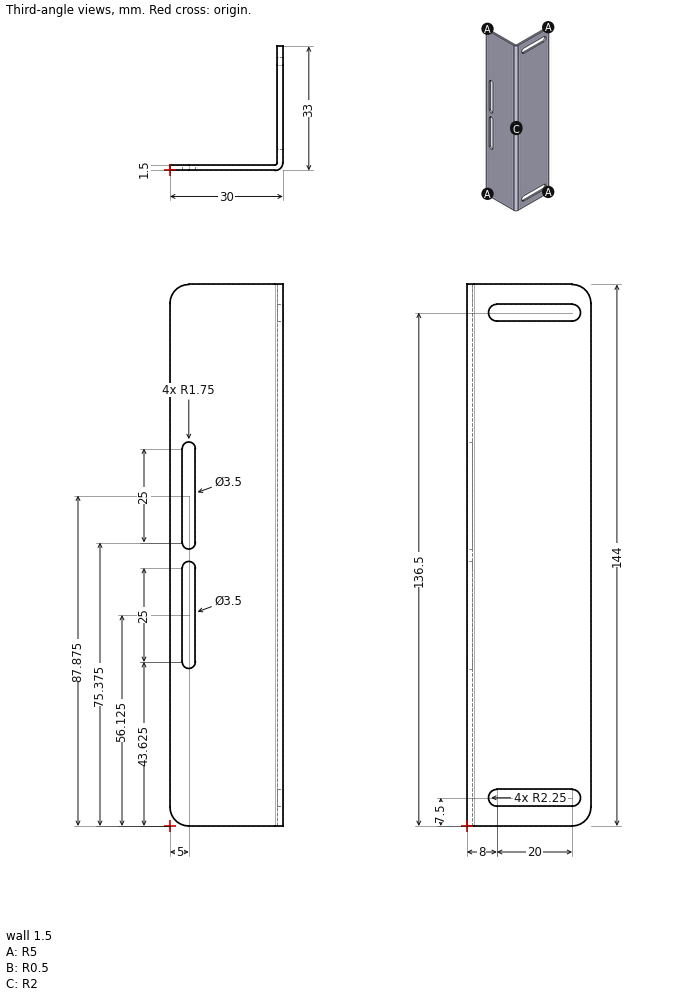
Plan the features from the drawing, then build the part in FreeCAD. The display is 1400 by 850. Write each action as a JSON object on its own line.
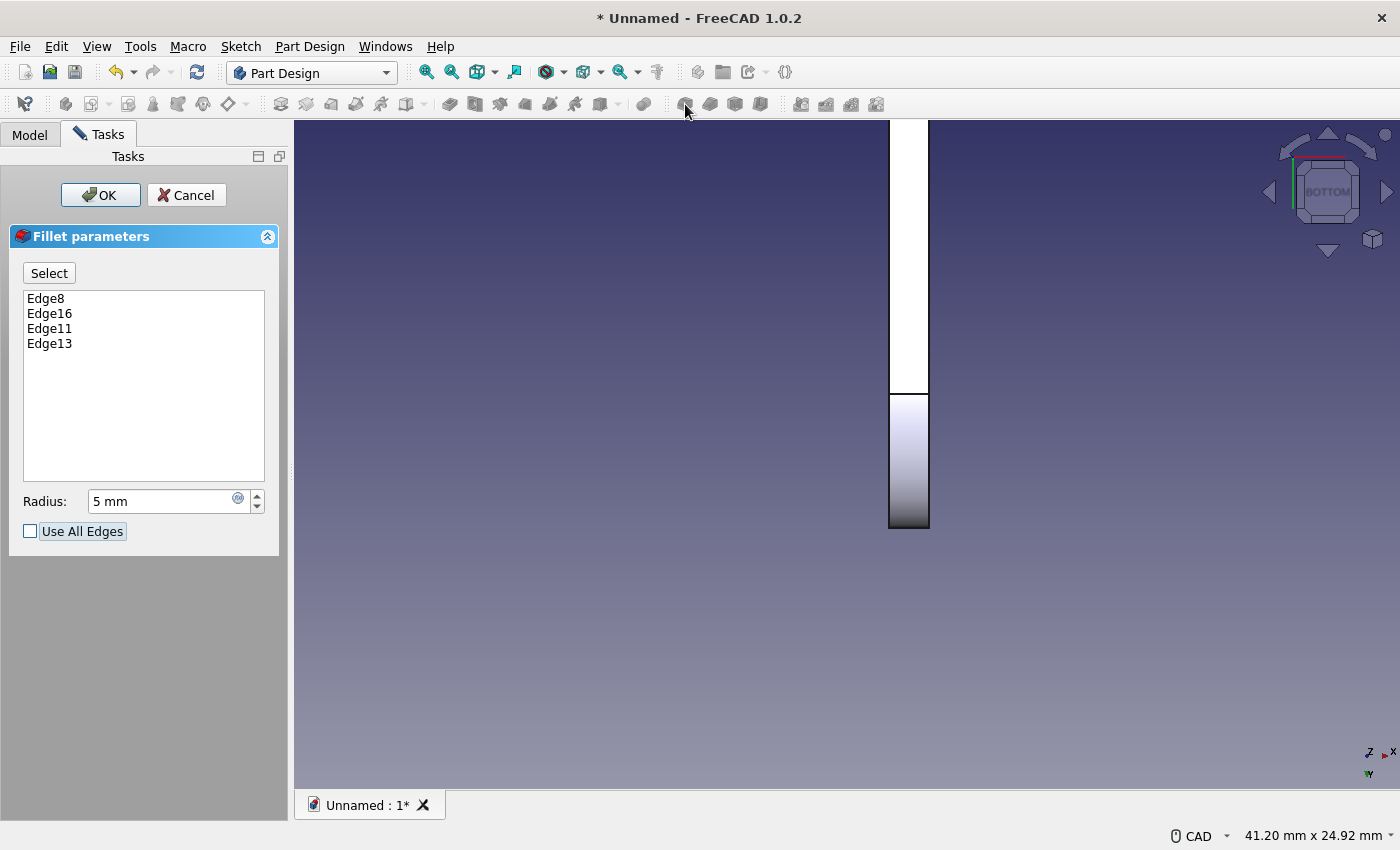
{"action": "left_click", "coordinate": [101, 195]}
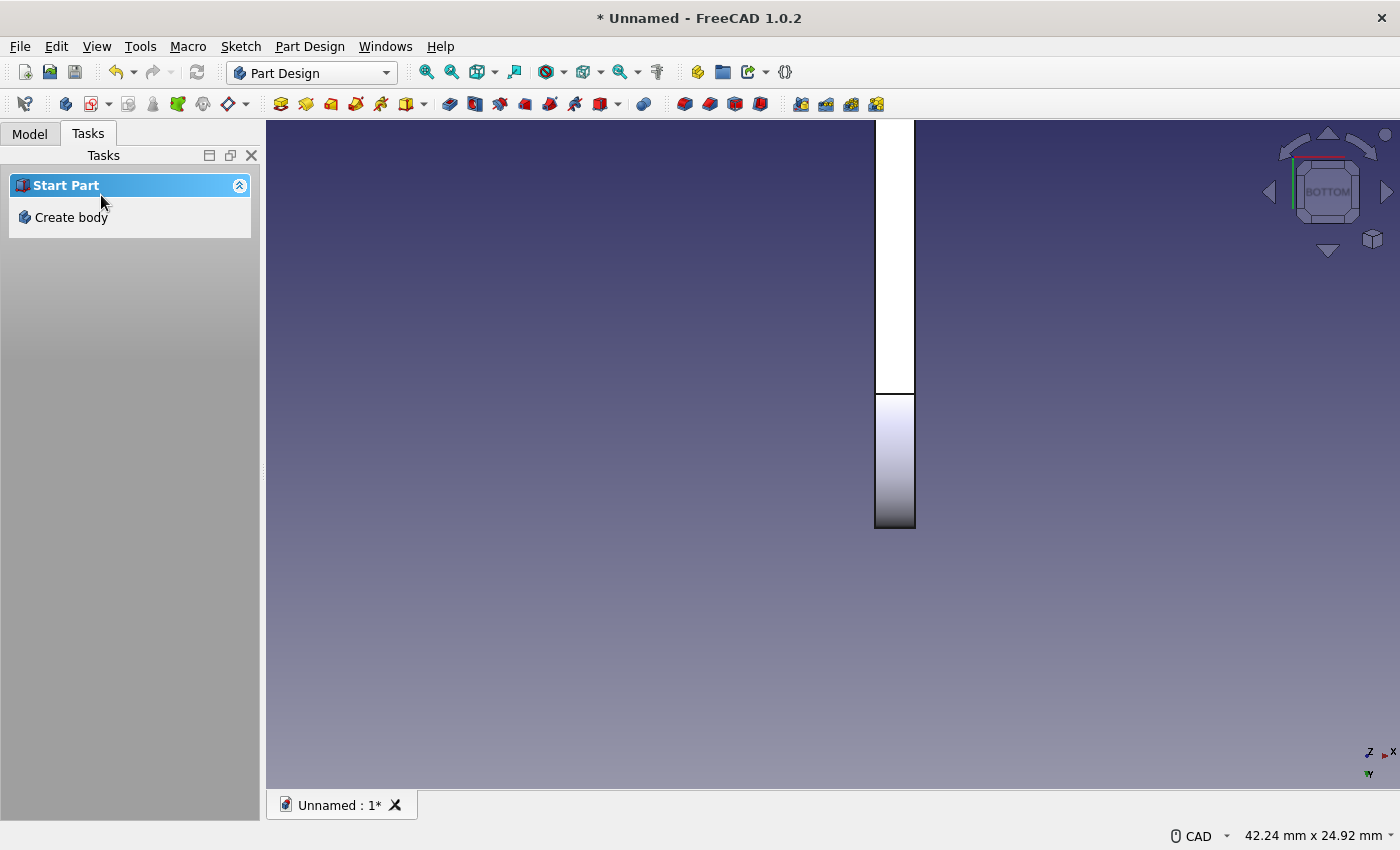
{"action": "left_click", "coordinate": [427, 72]}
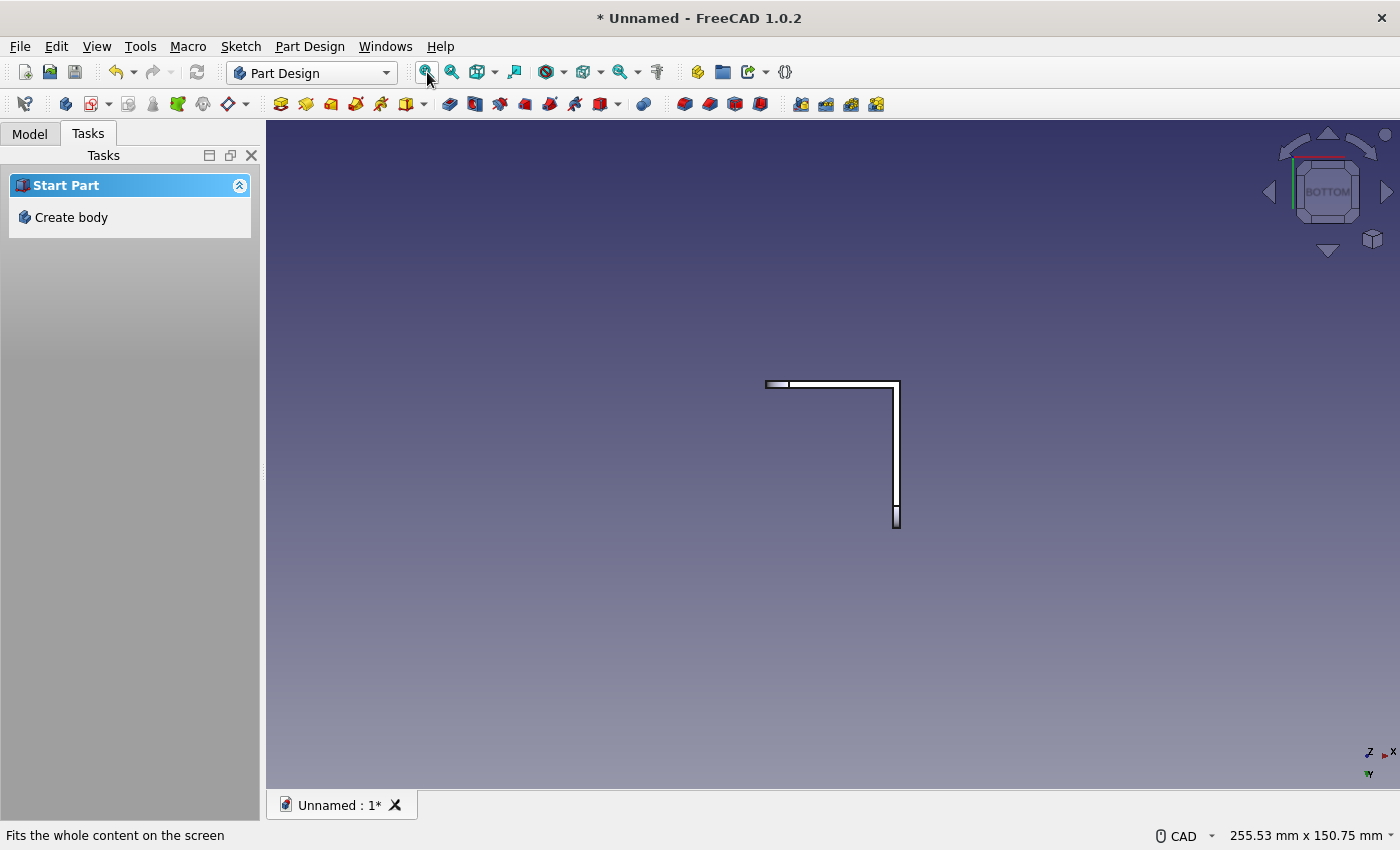
{"action": "key", "text": "0"}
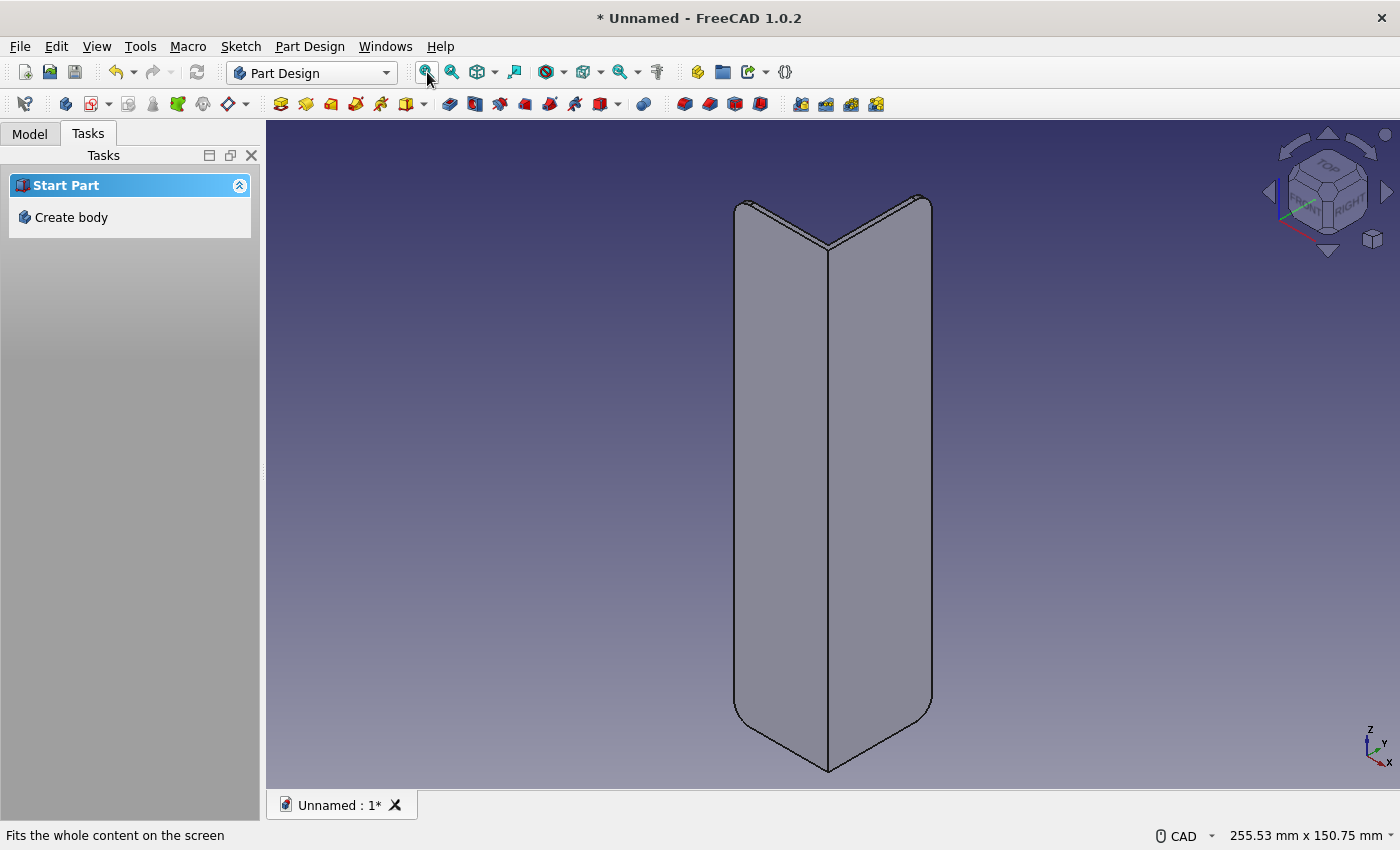
{"action": "key", "text": "2"}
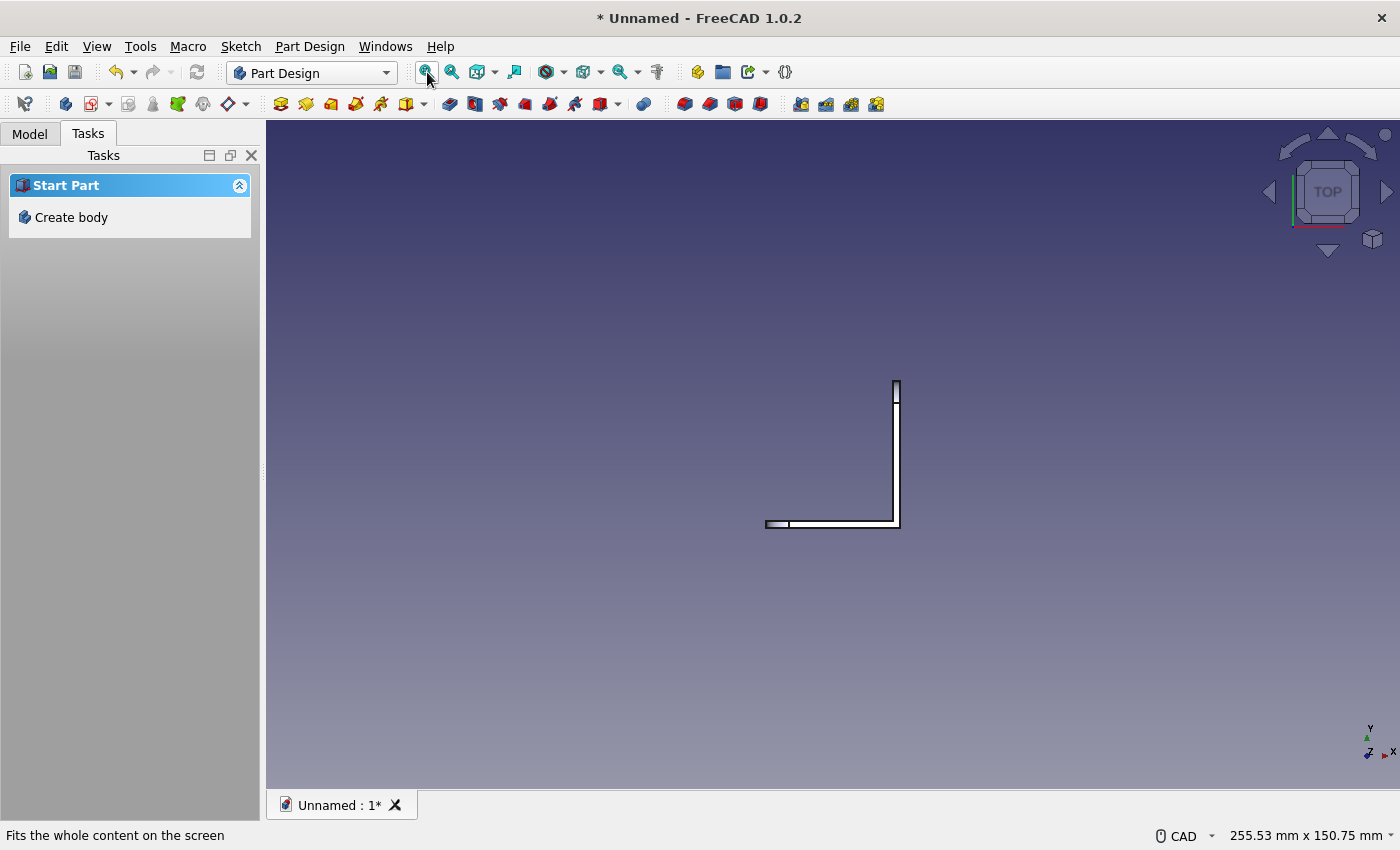
{"action": "left_click", "coordinate": [427, 72]}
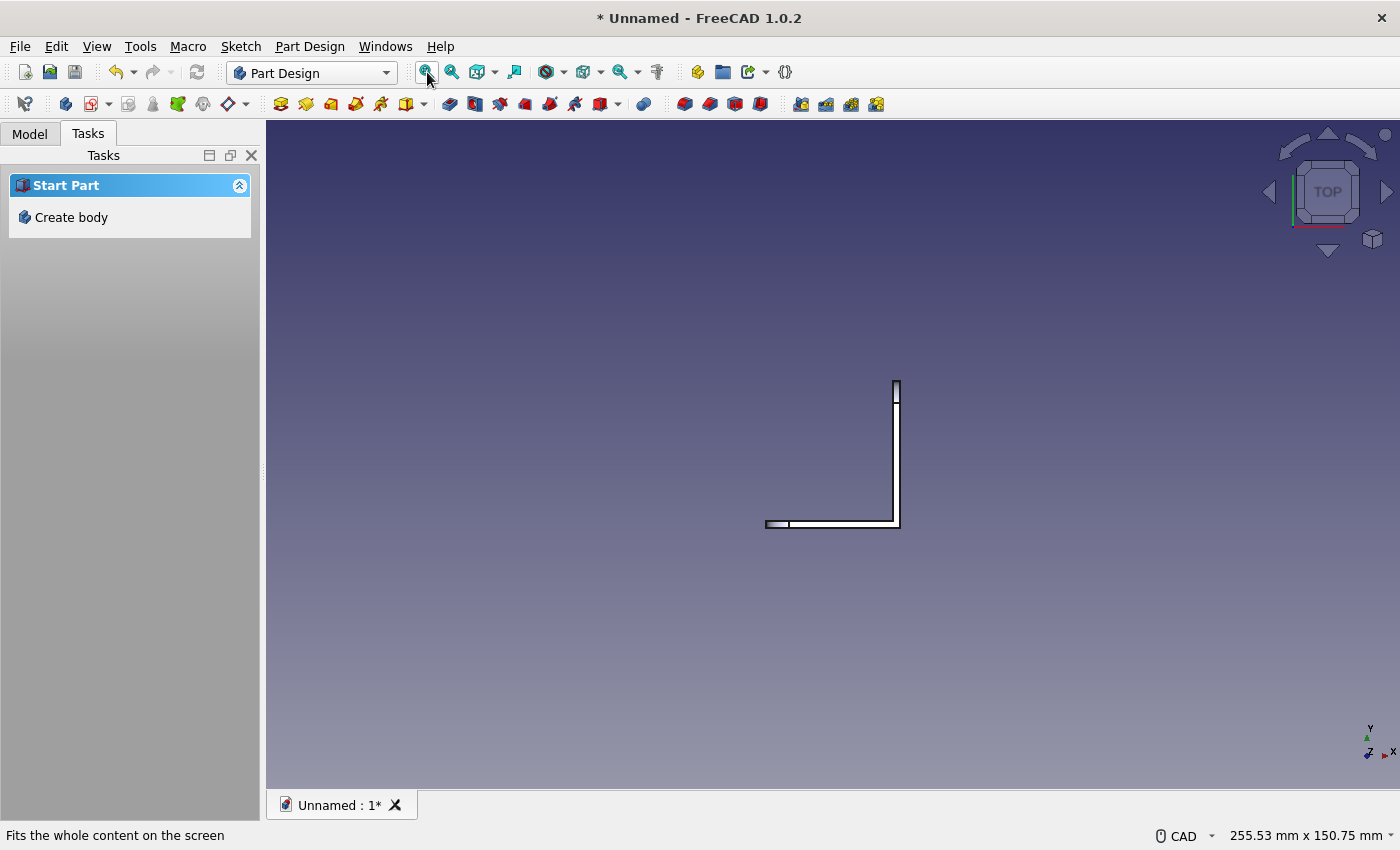
{"action": "key", "text": "1"}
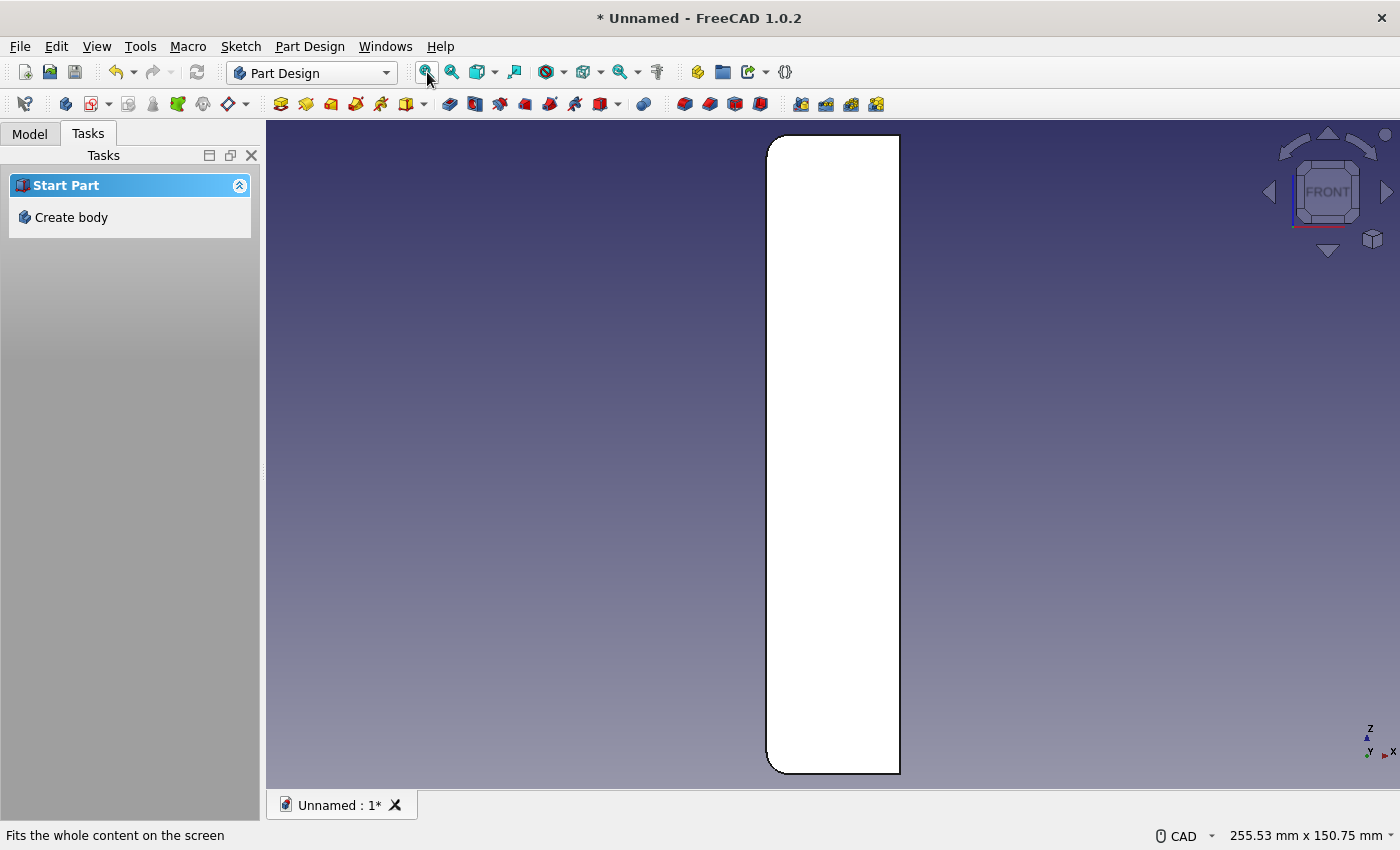
{"action": "key", "text": "3"}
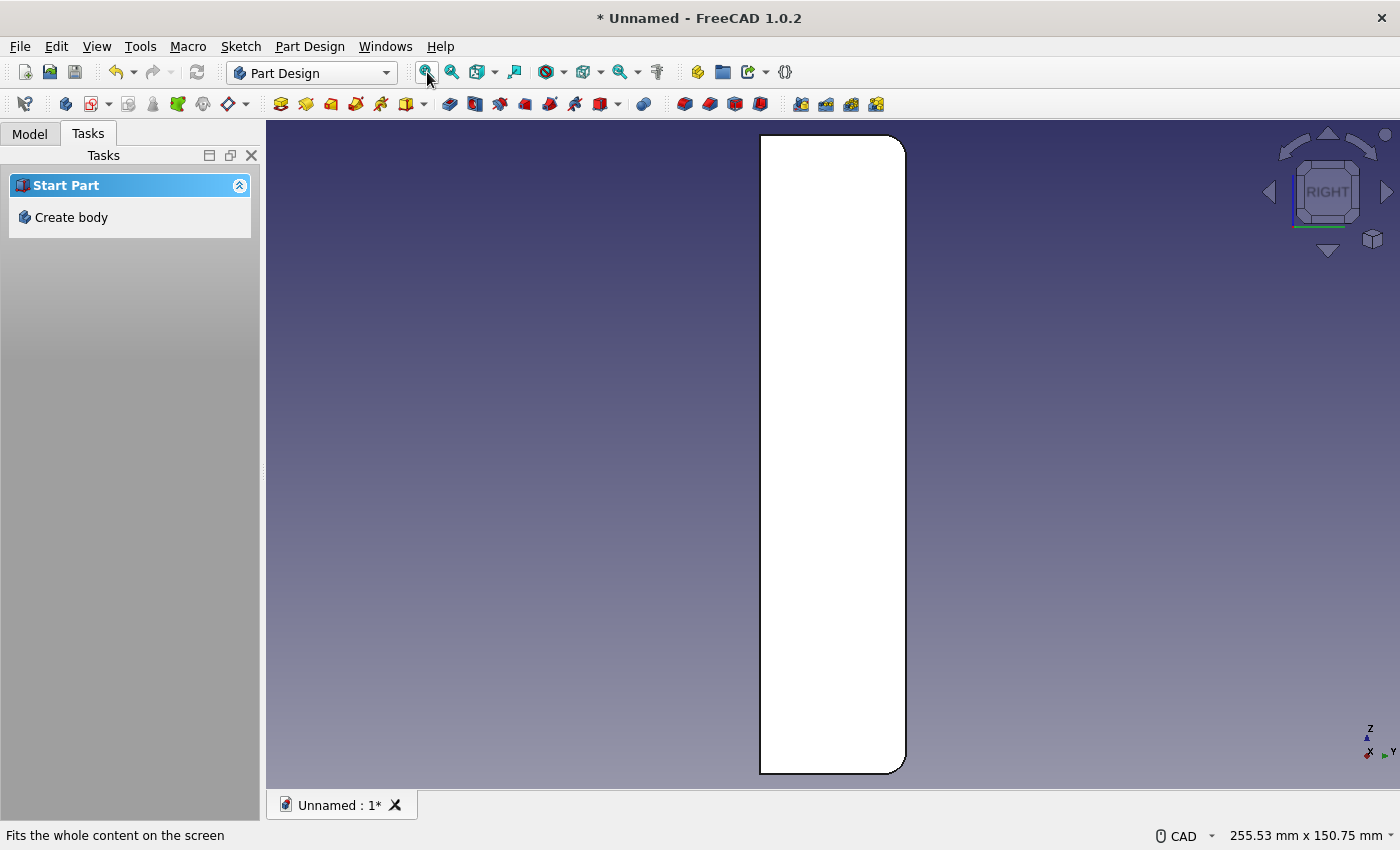
{"action": "key", "text": "5"}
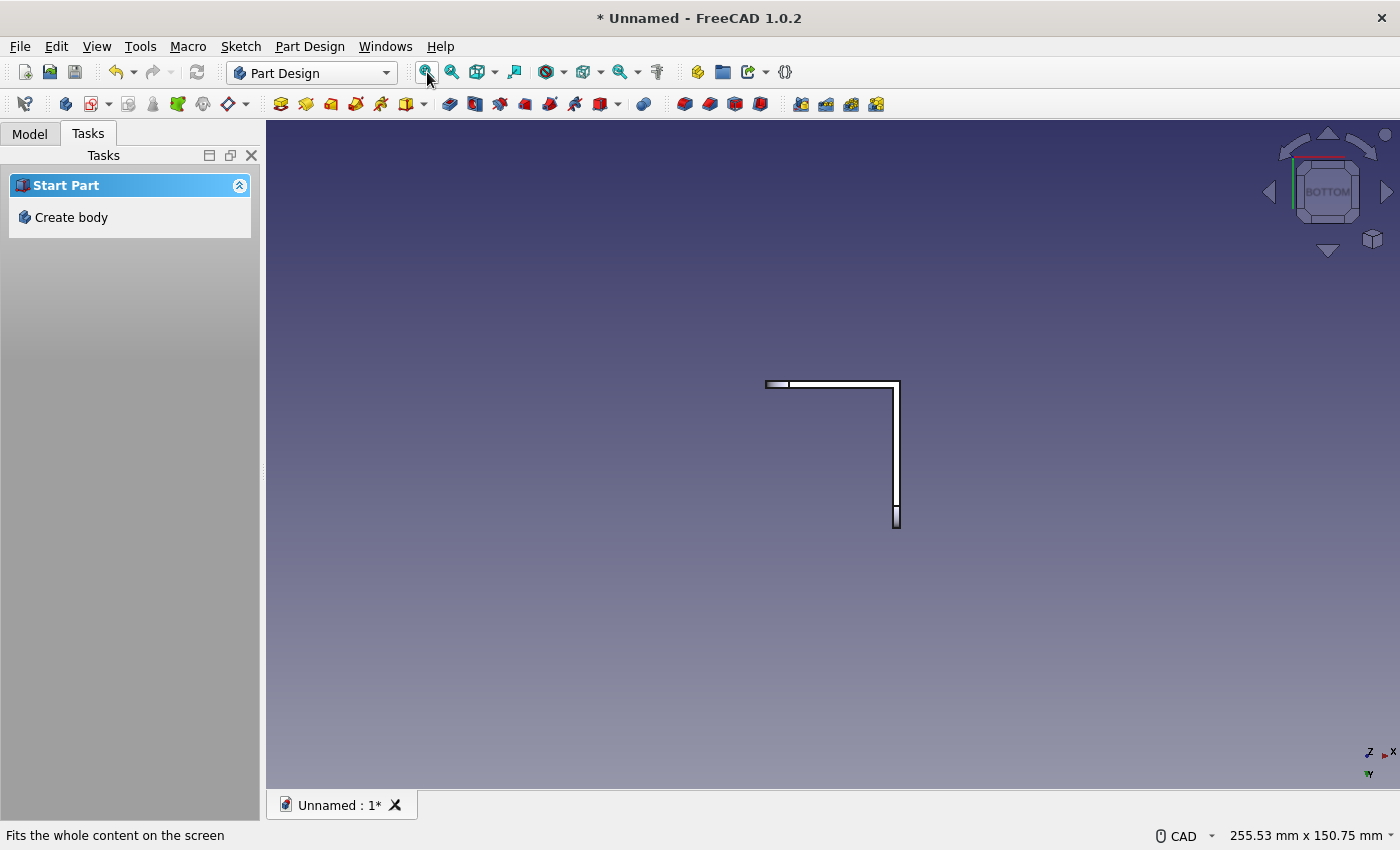
{"action": "left_click", "coordinate": [427, 72]}